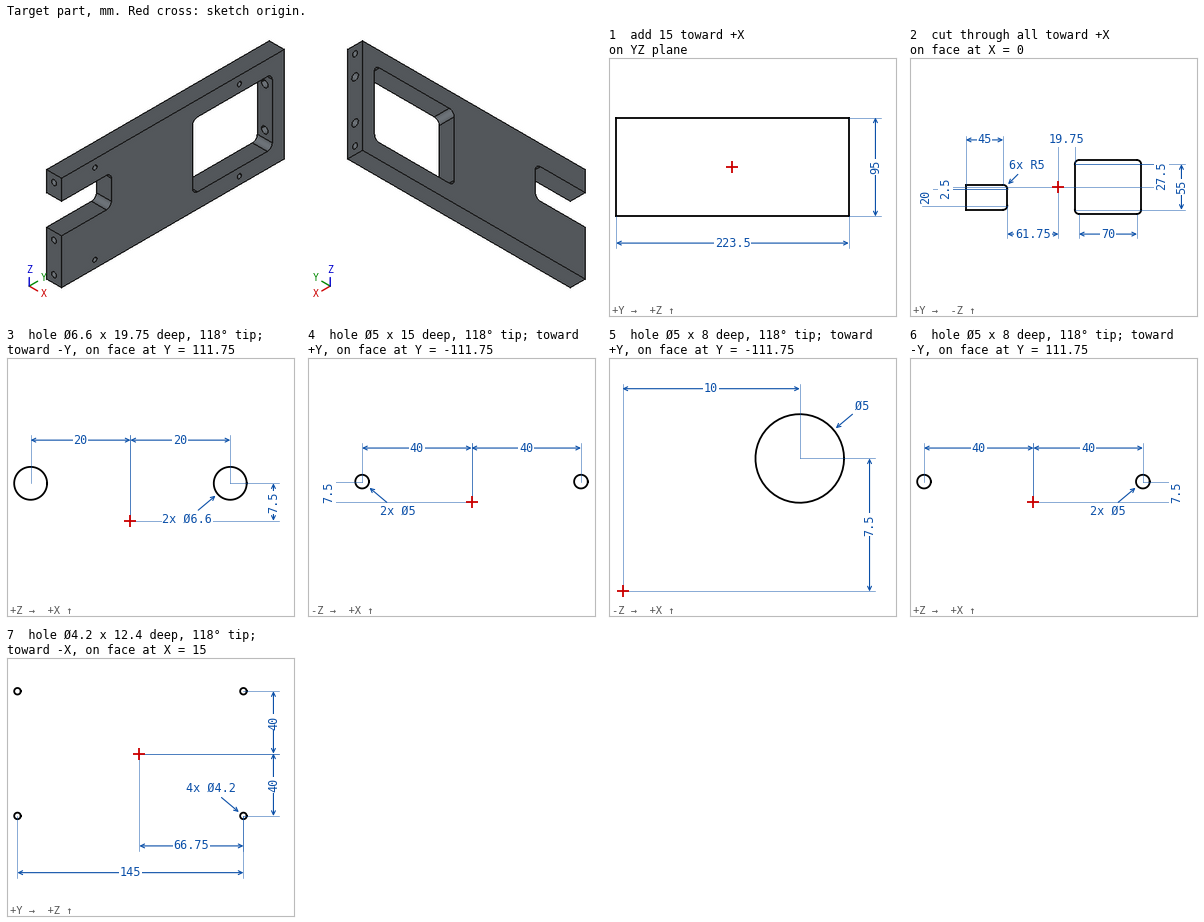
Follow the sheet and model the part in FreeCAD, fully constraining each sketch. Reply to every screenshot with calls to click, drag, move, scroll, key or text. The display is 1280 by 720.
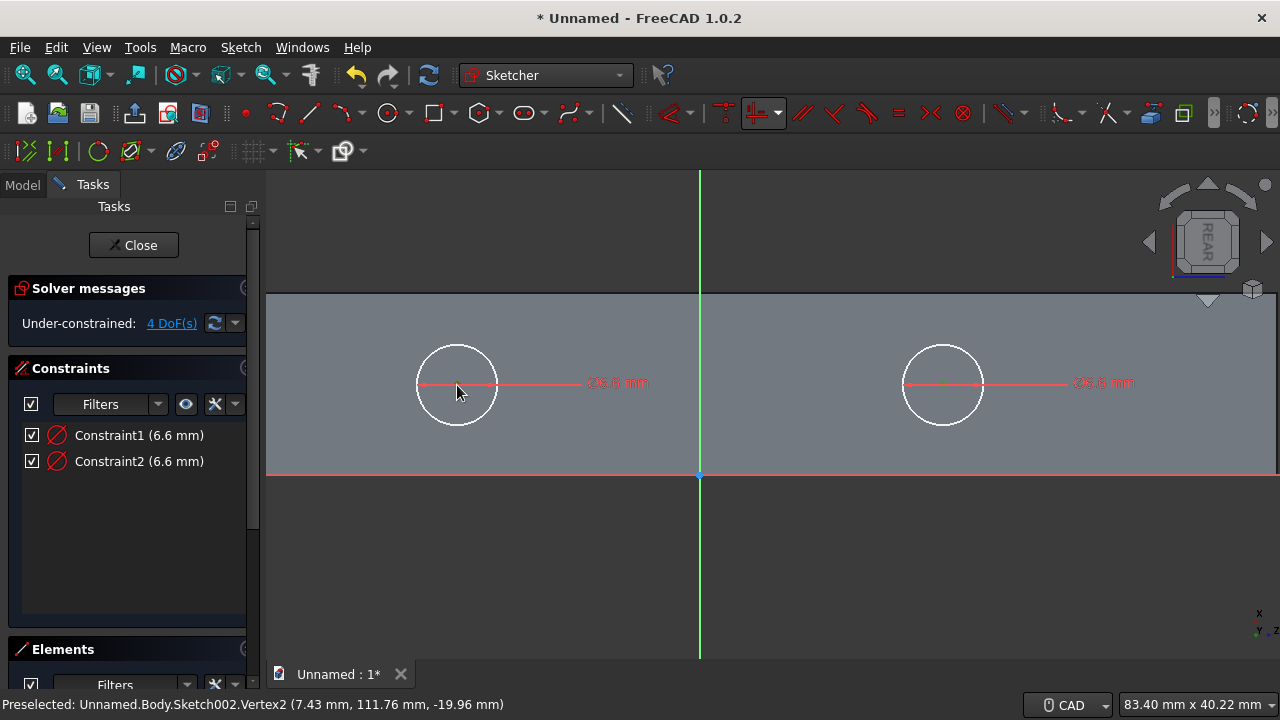
key(h)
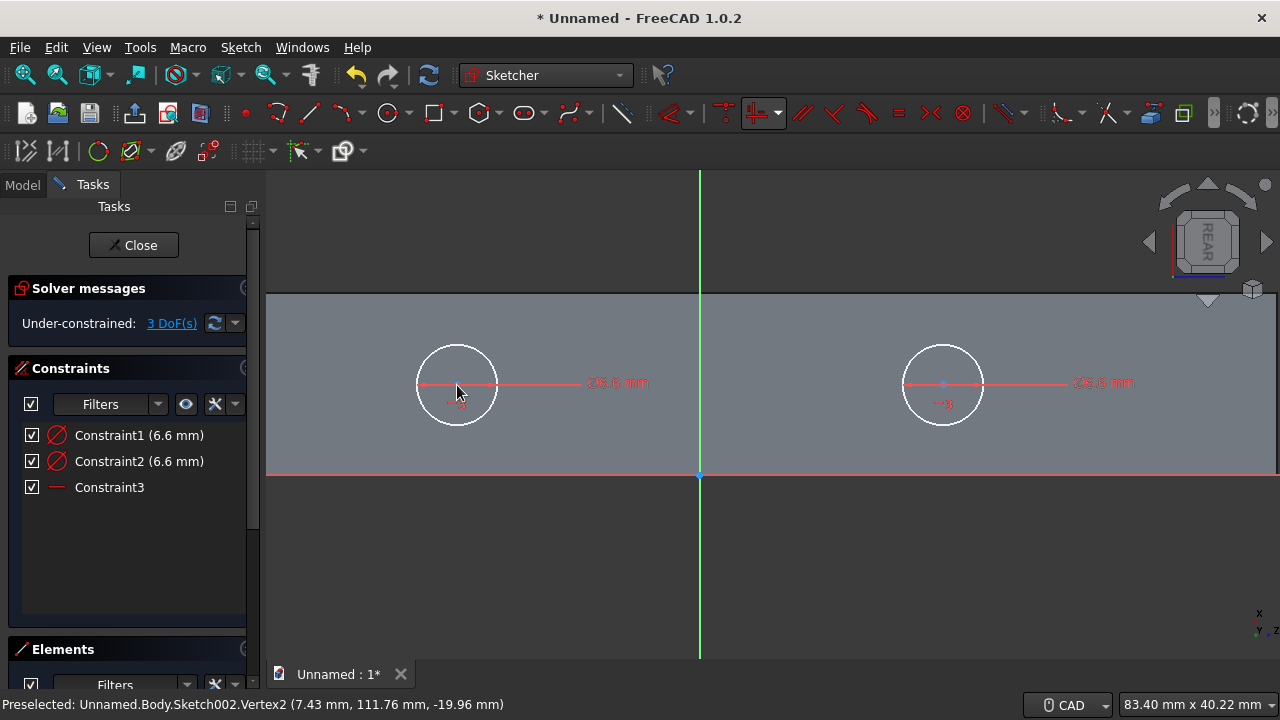
click(670, 114)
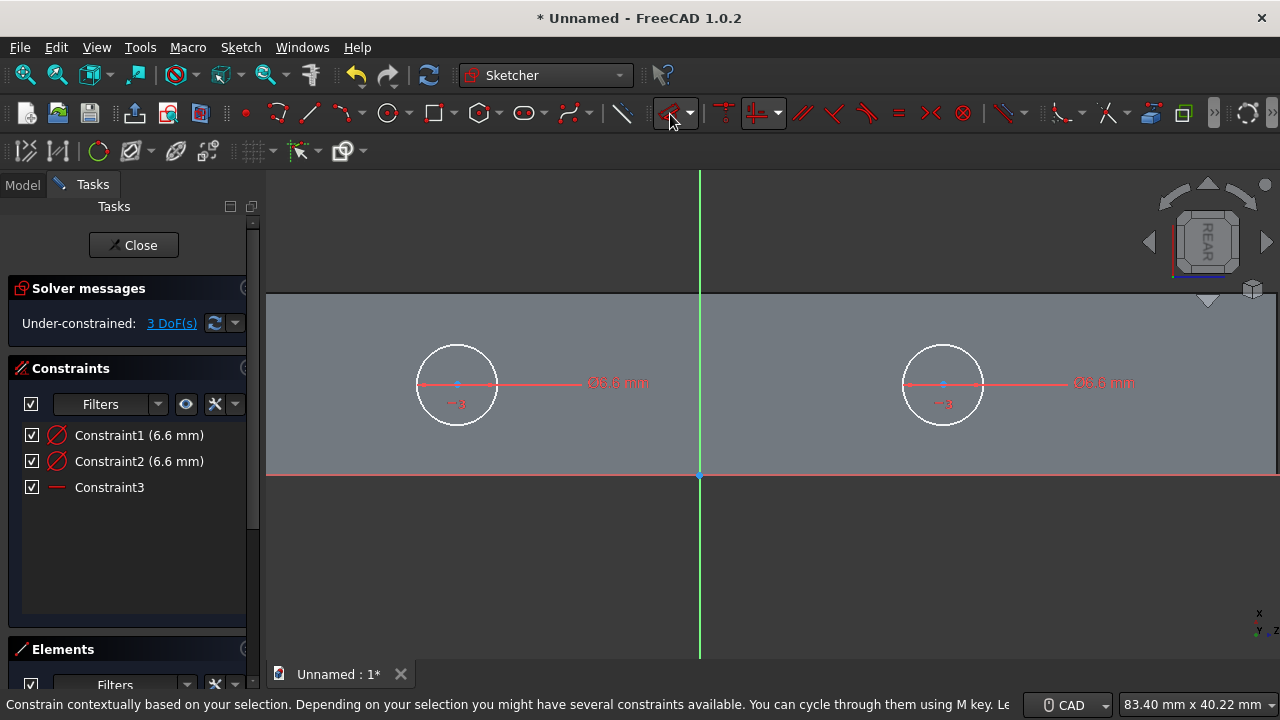
click(943, 385)
click(821, 509)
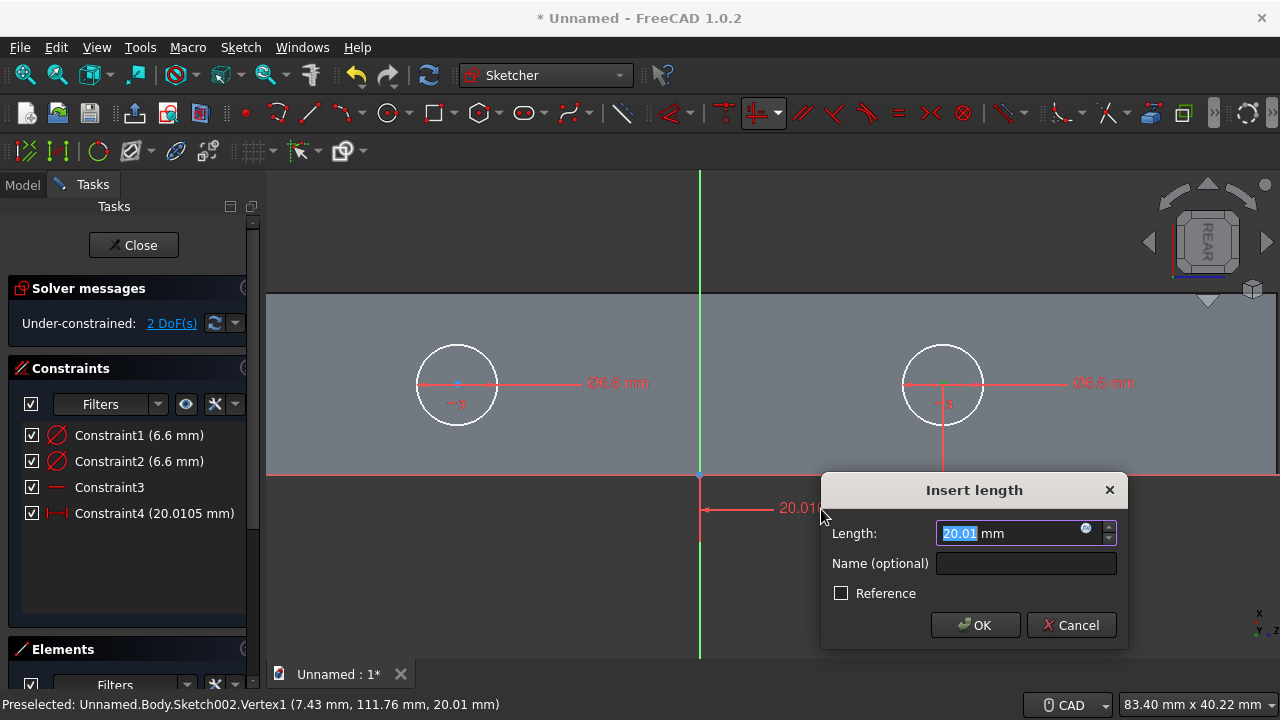
text(20)
key(Return)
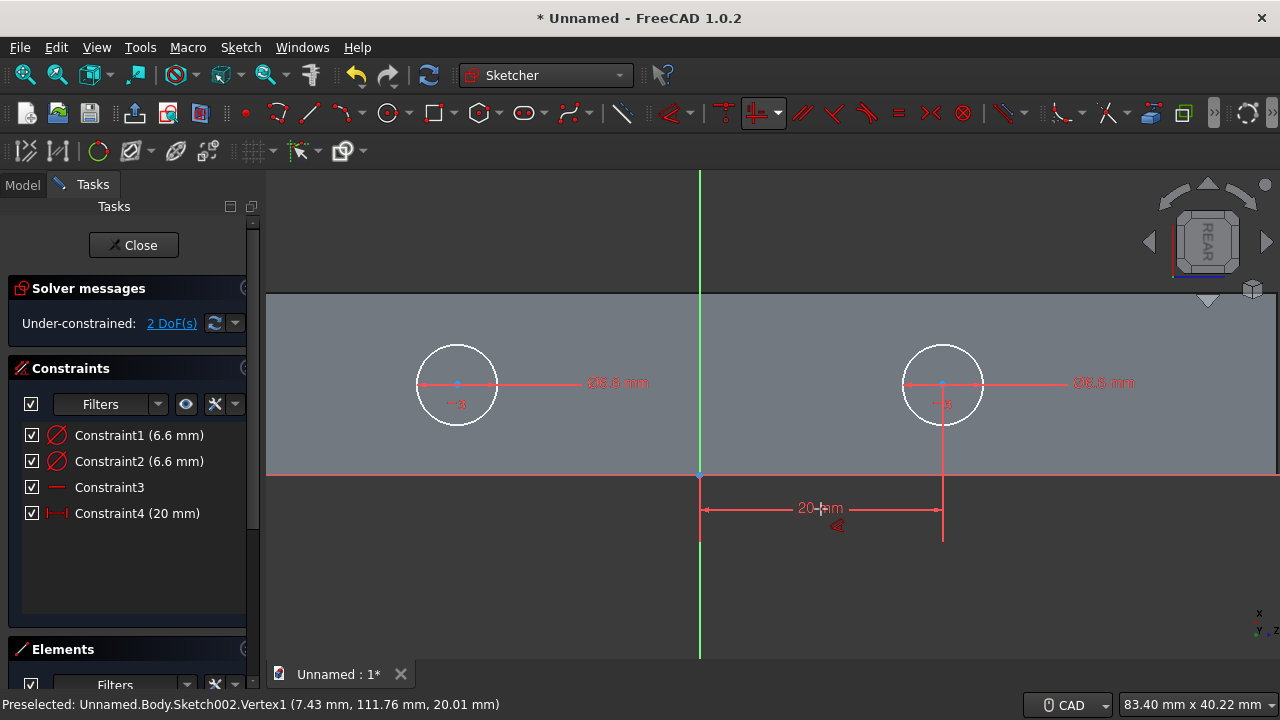
click(457, 385)
click(578, 509)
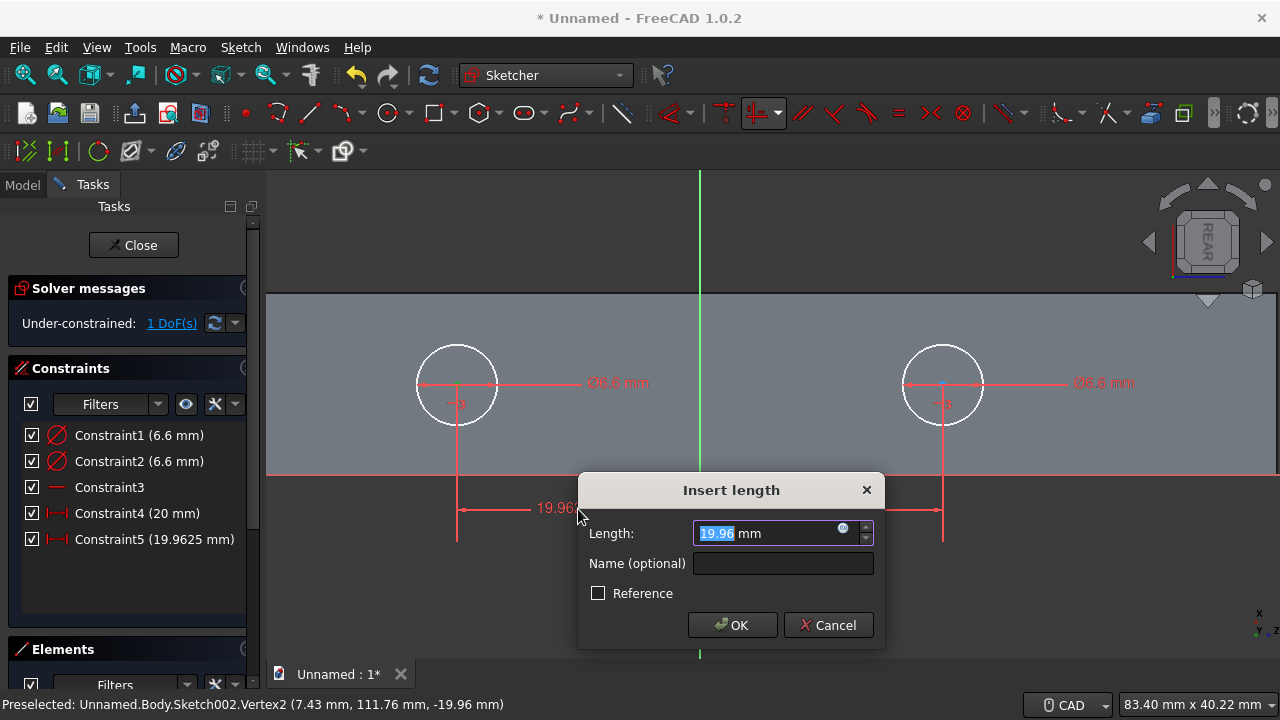
text(20)
key(Return)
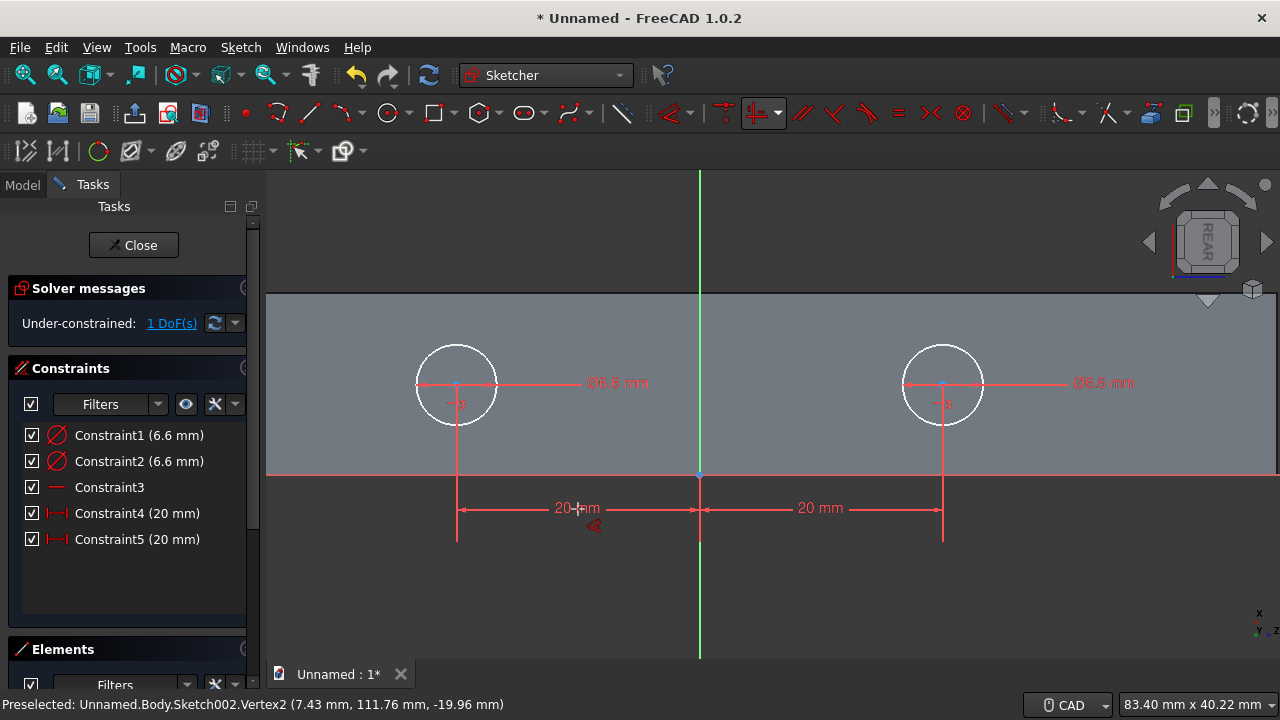
click(943, 385)
click(977, 430)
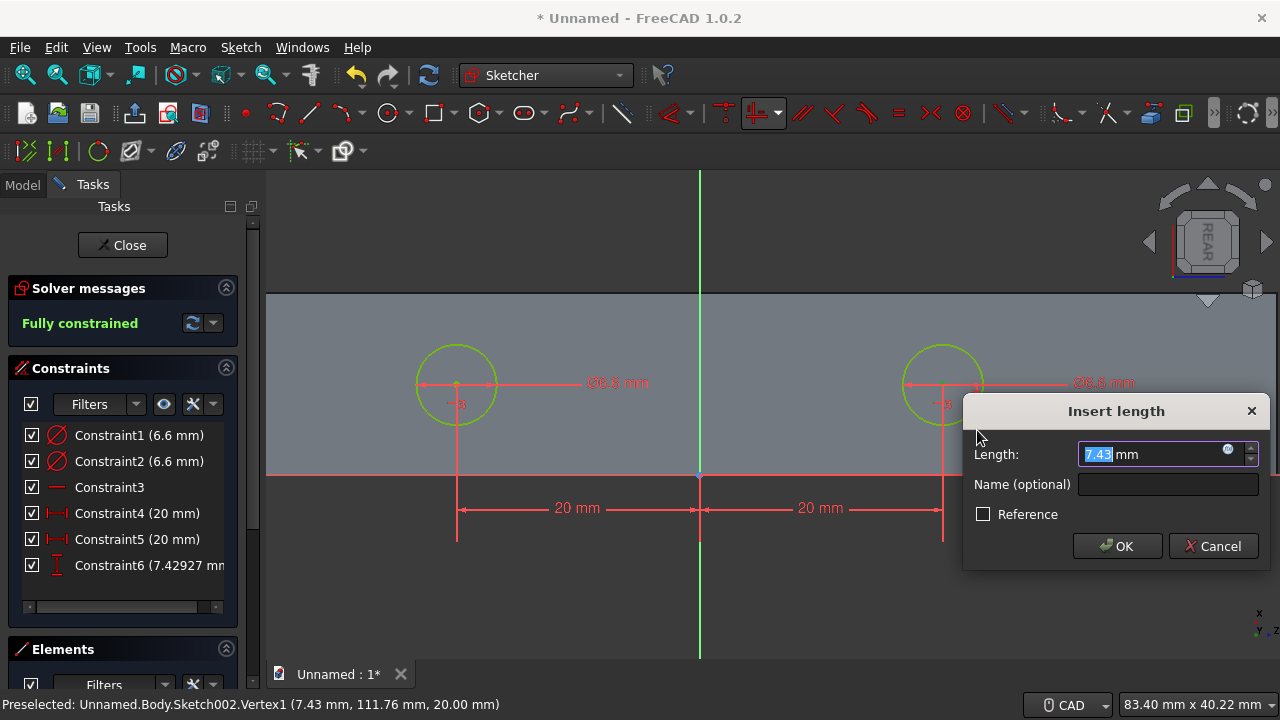
text(7.5)
key(Return)
key(Escape)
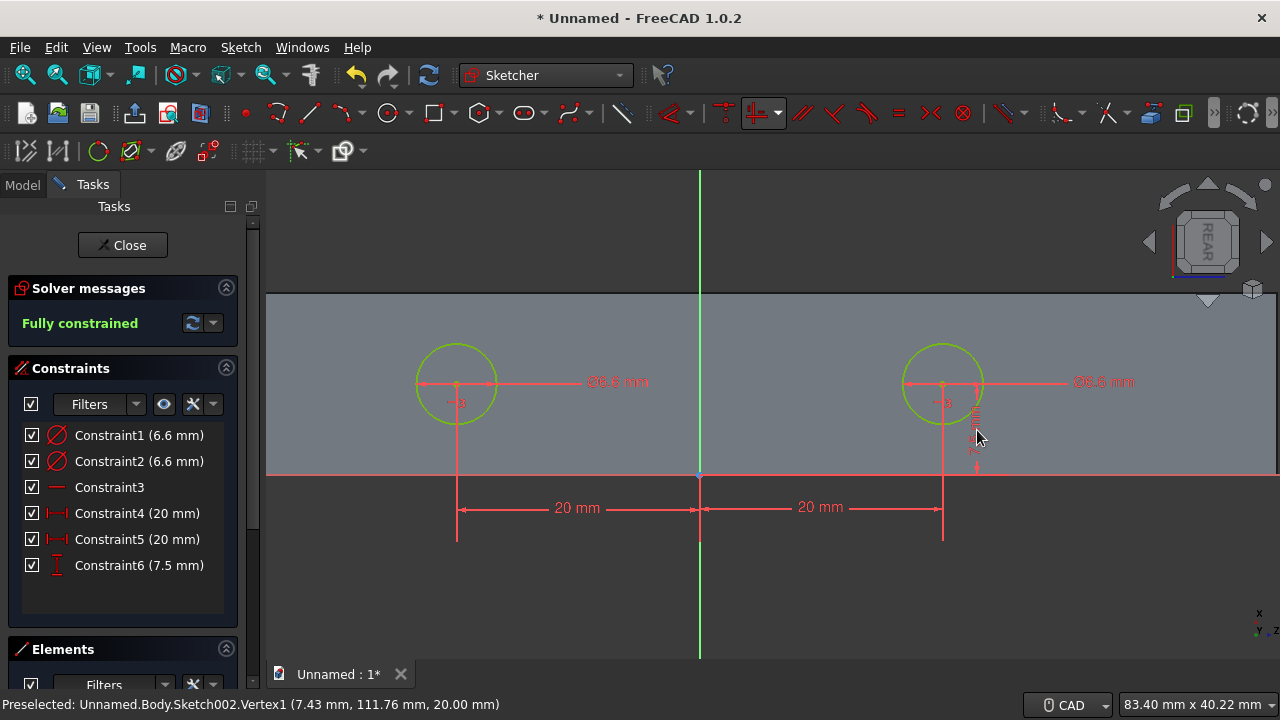
click(123, 245)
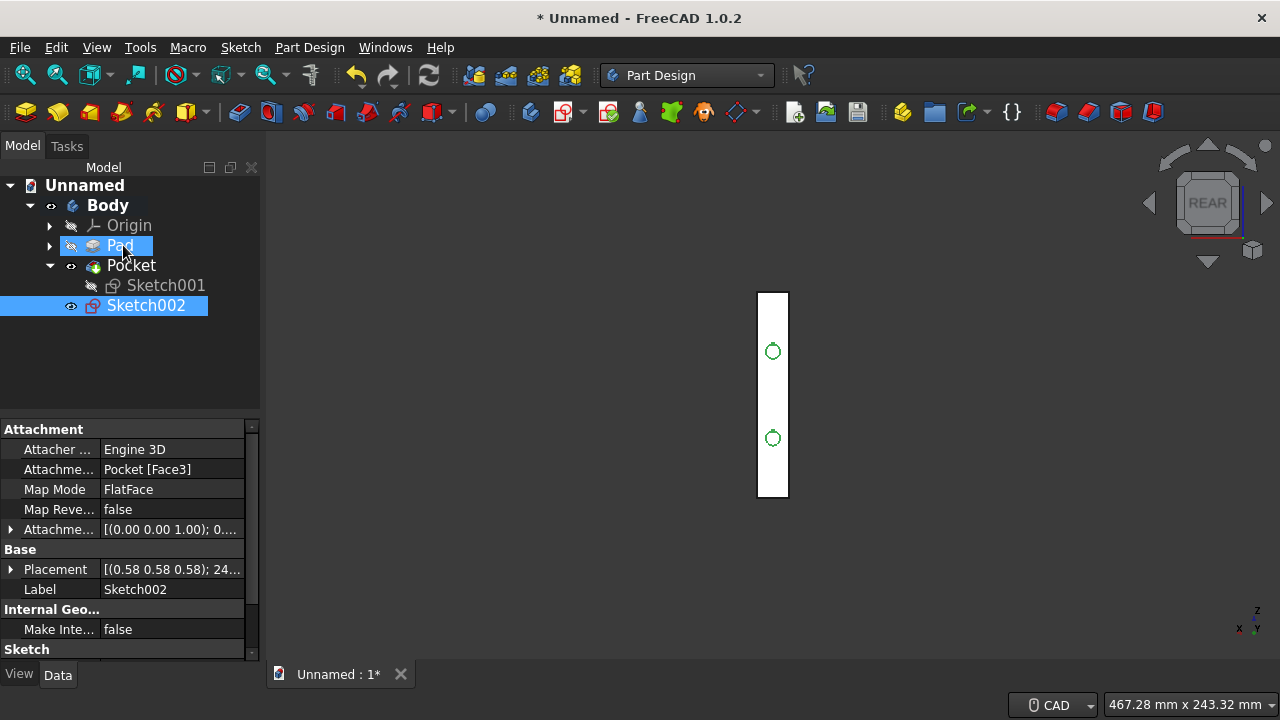
click(272, 112)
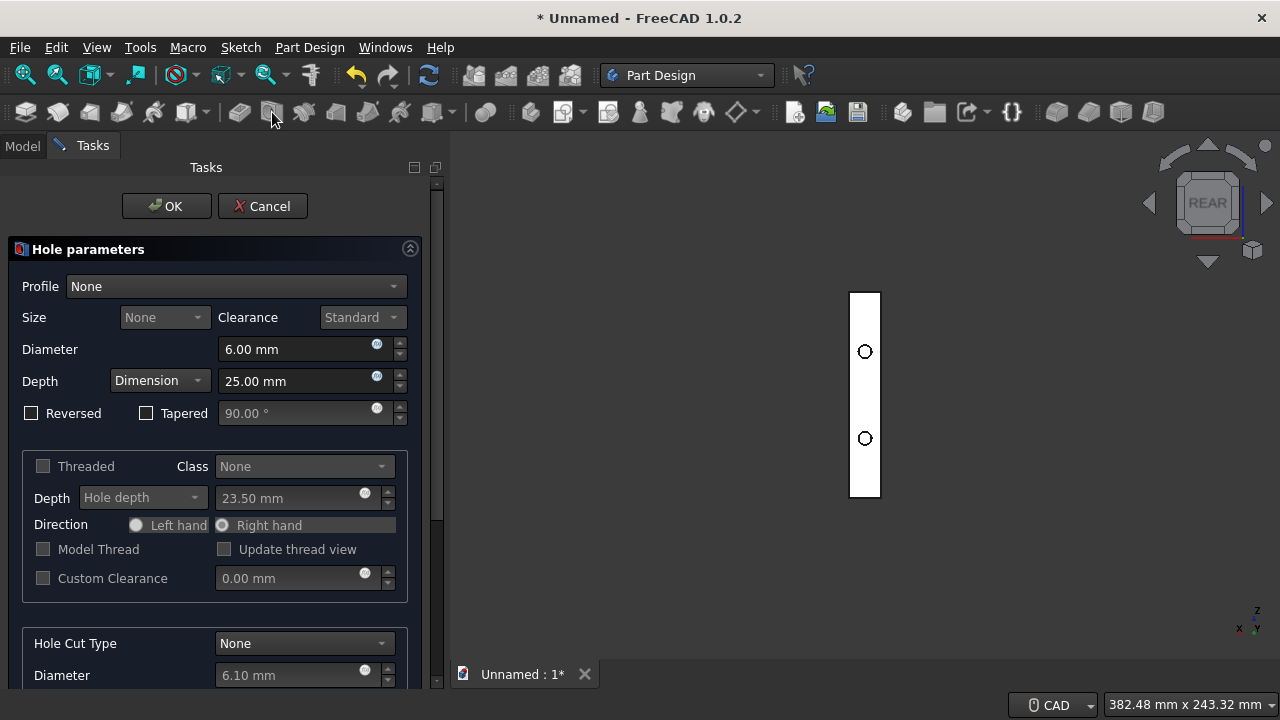
triple_click(305, 349)